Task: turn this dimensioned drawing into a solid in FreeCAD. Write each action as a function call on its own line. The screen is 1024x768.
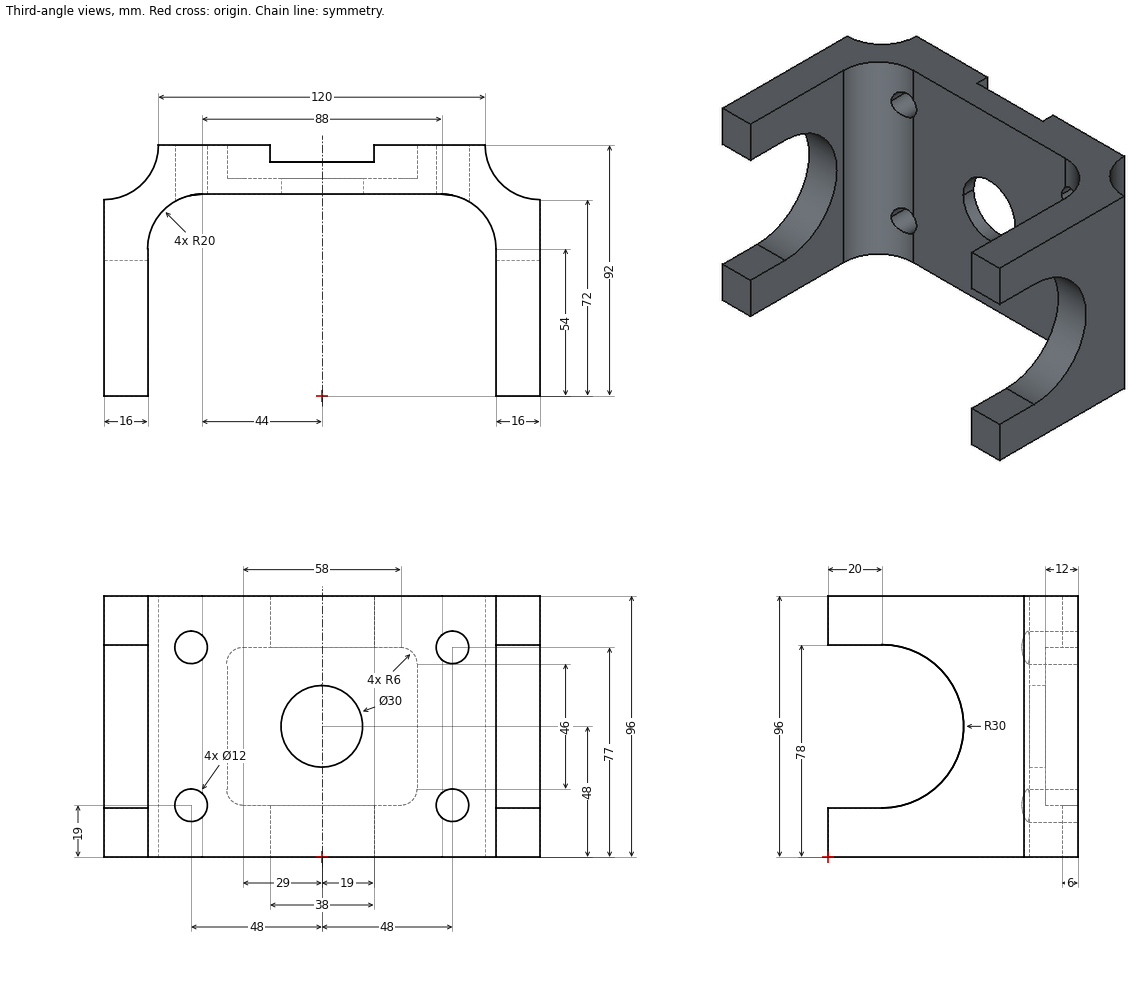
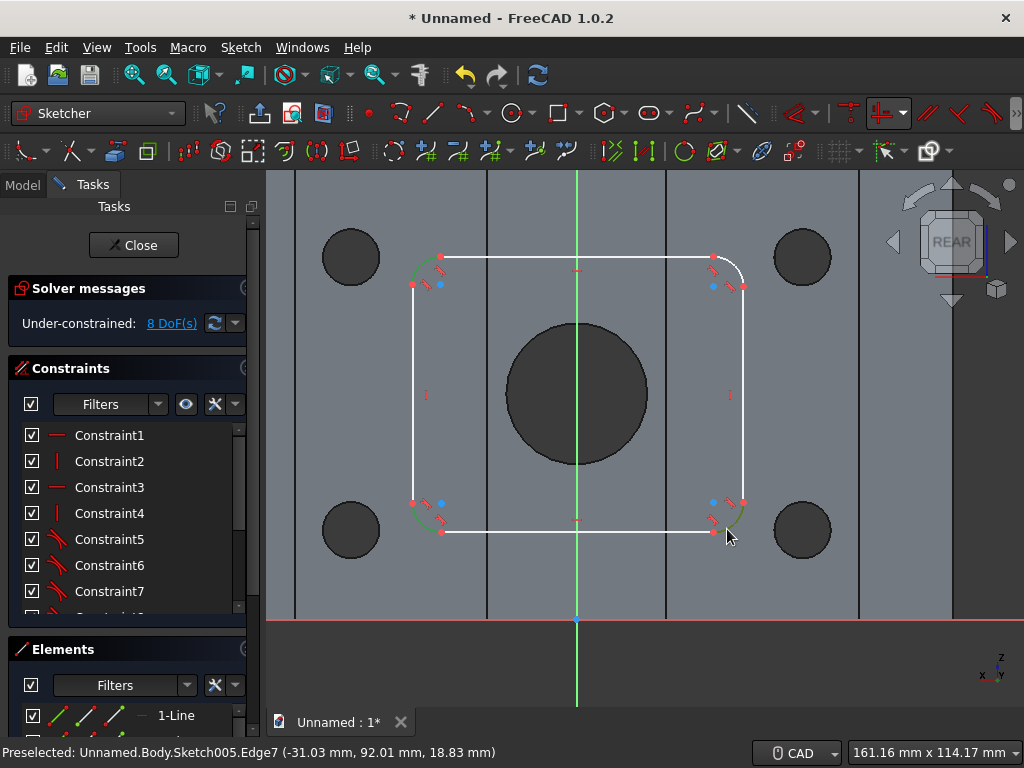
click(740, 273)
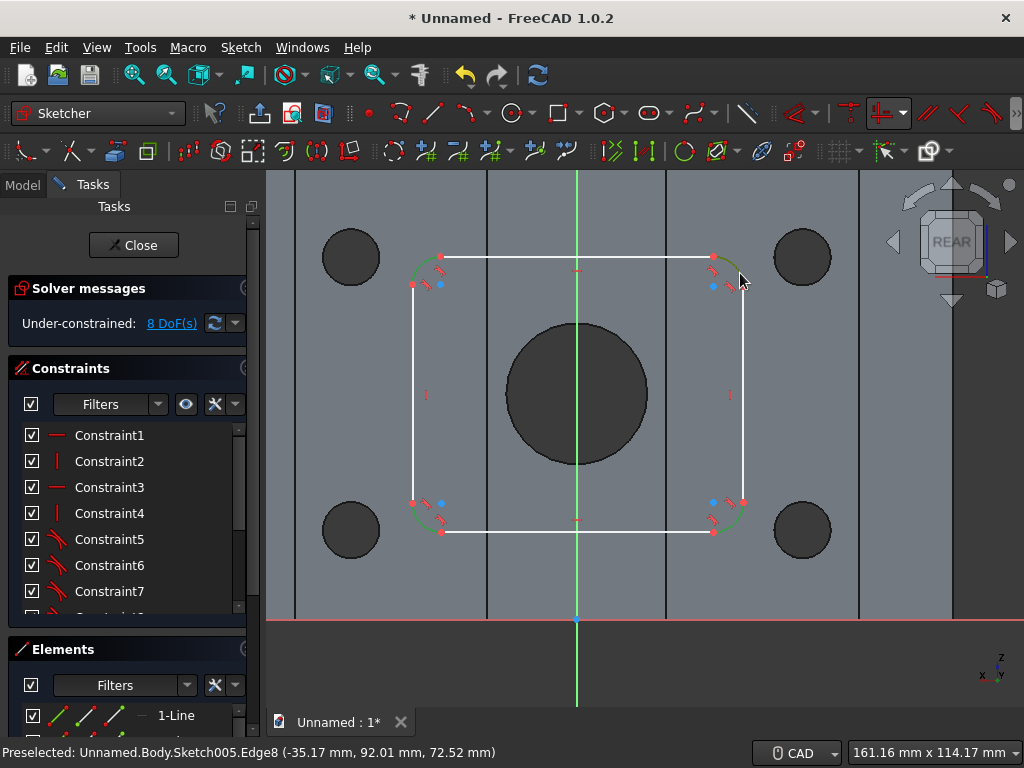
key(e)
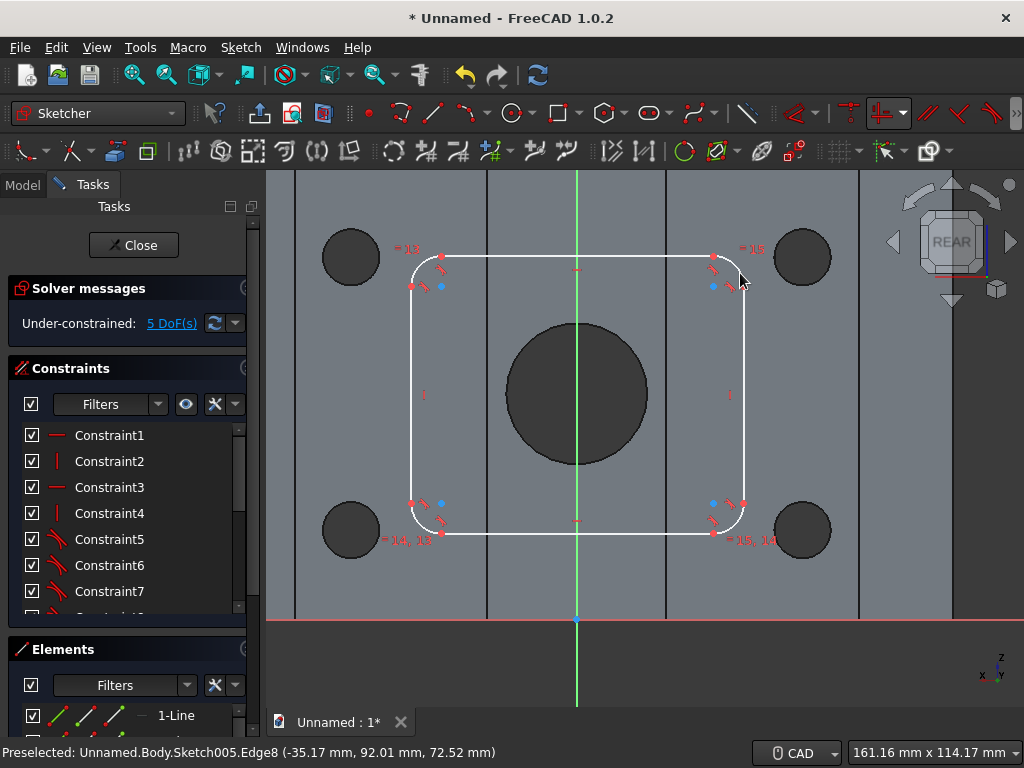
click(794, 114)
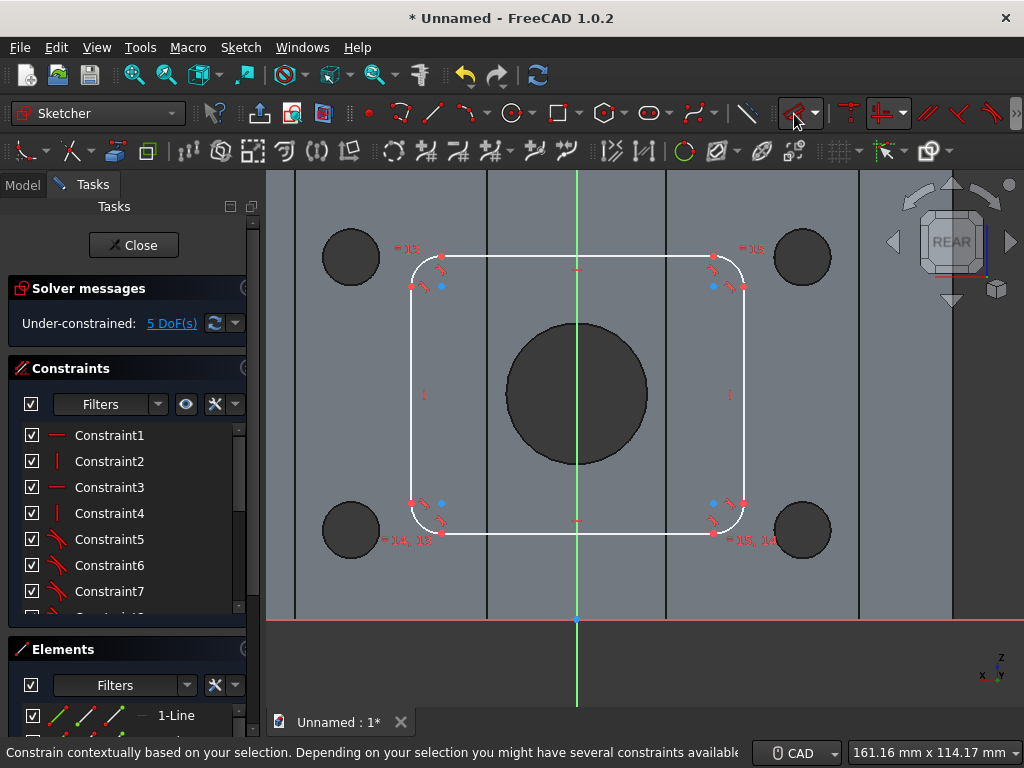
scroll(428, 259, up, 2)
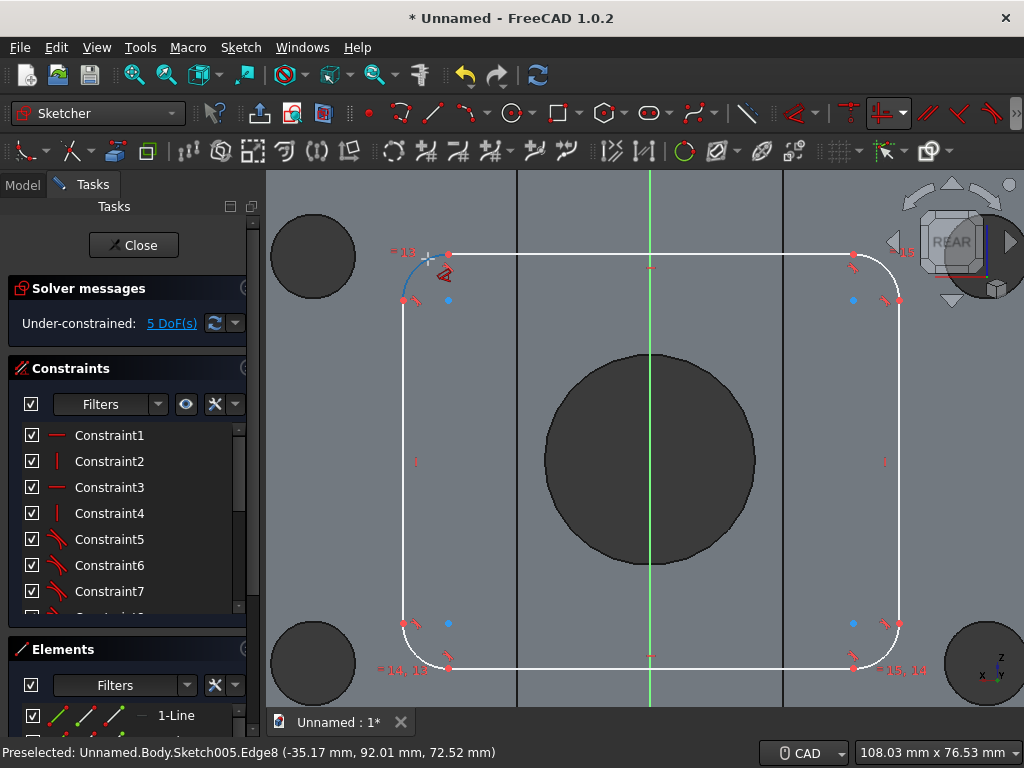
click(428, 259)
click(414, 230)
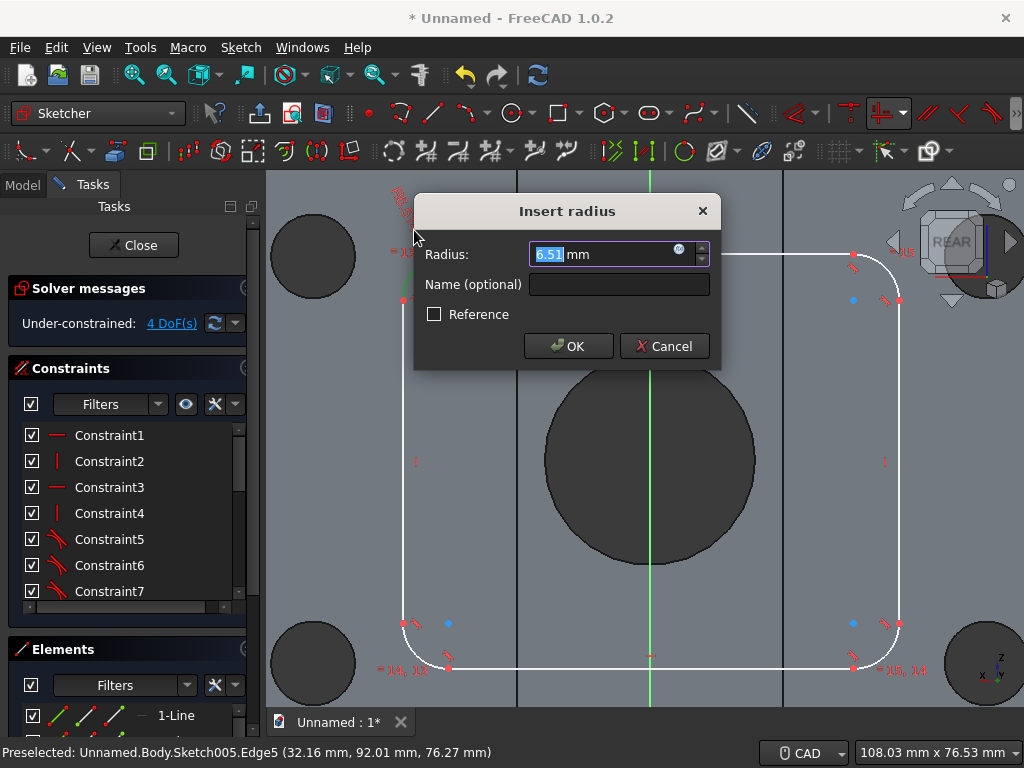
text(6)
key(Return)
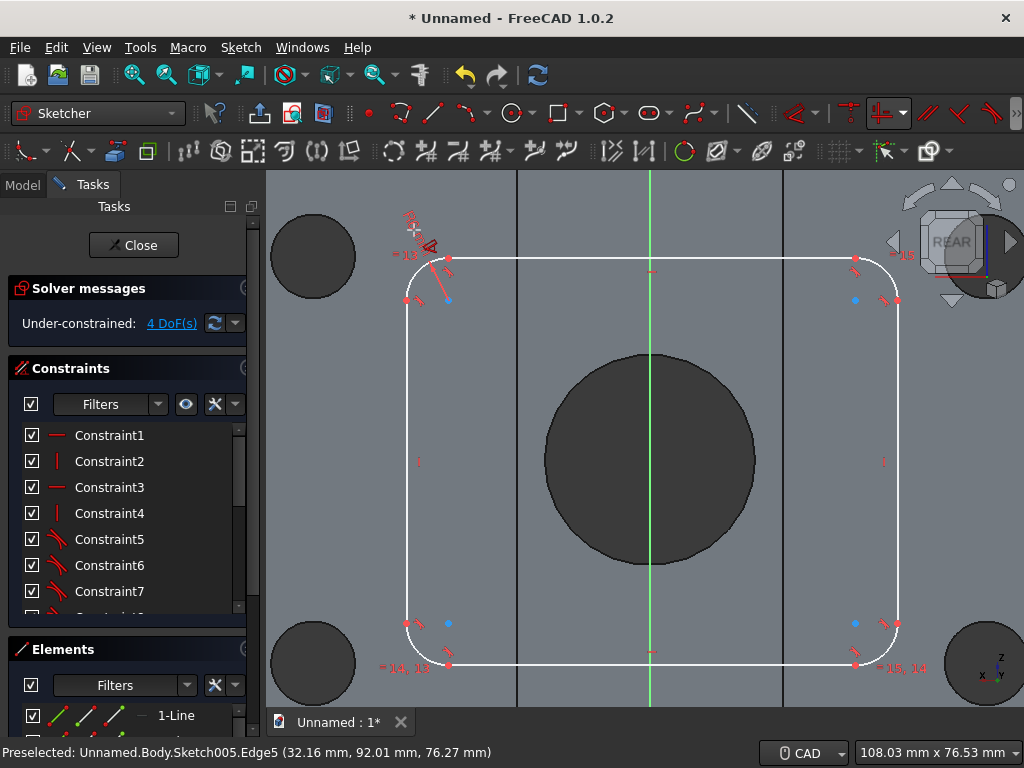
click(734, 258)
click(559, 224)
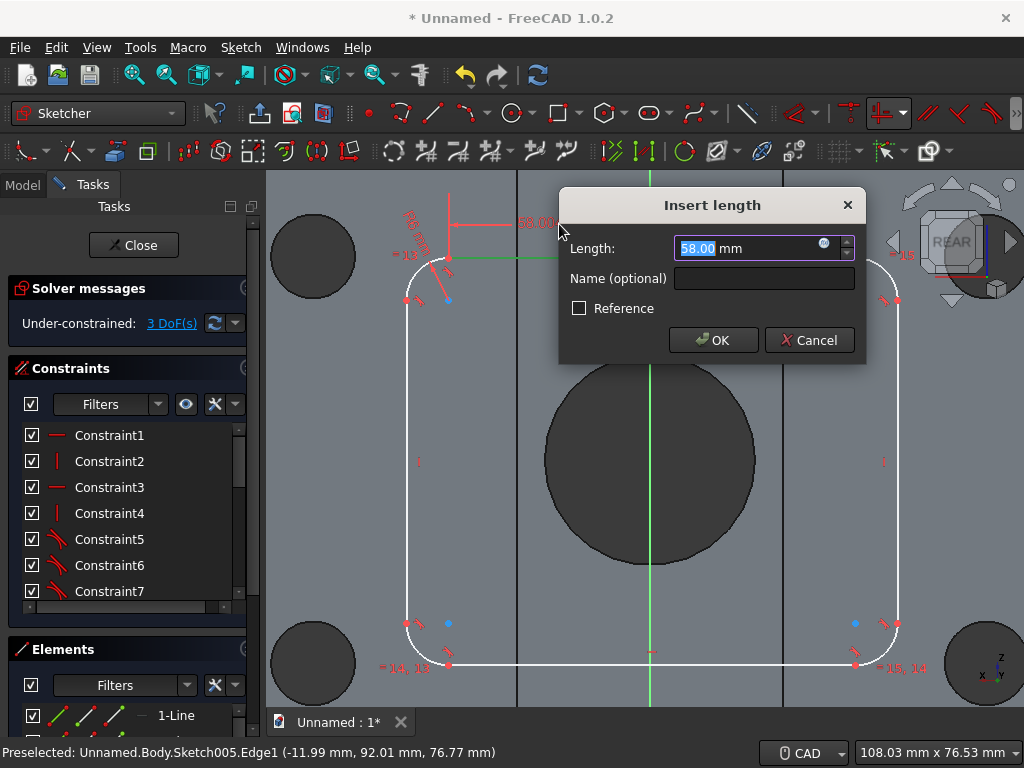
text(58)
key(Return)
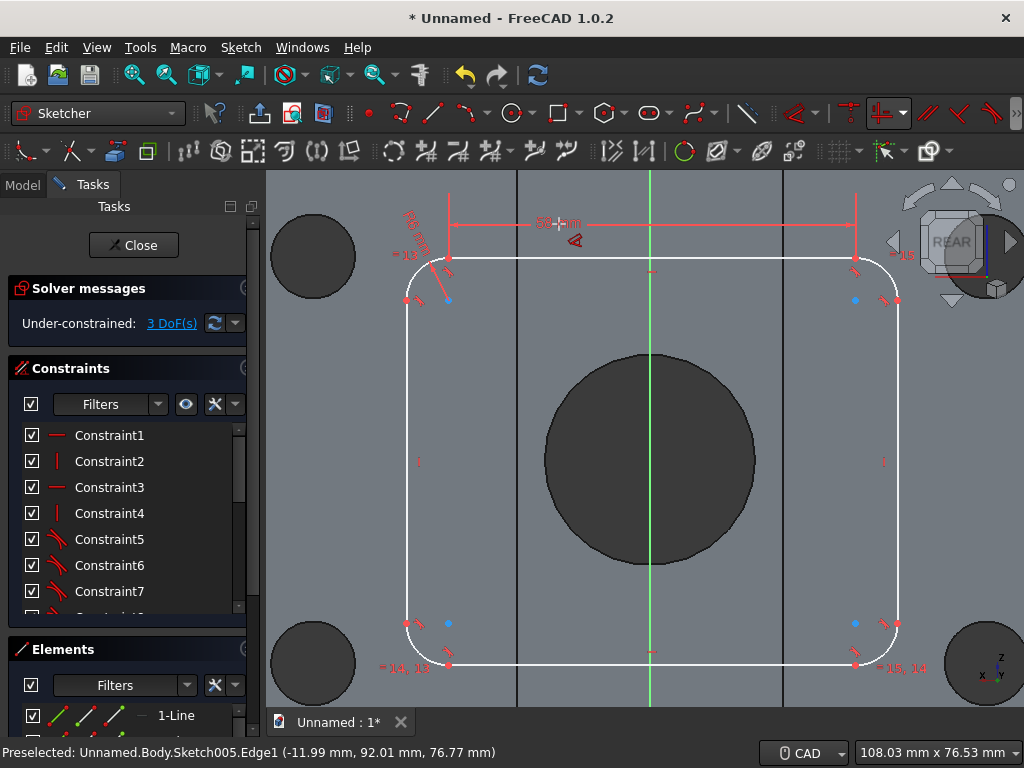
click(407, 397)
click(373, 462)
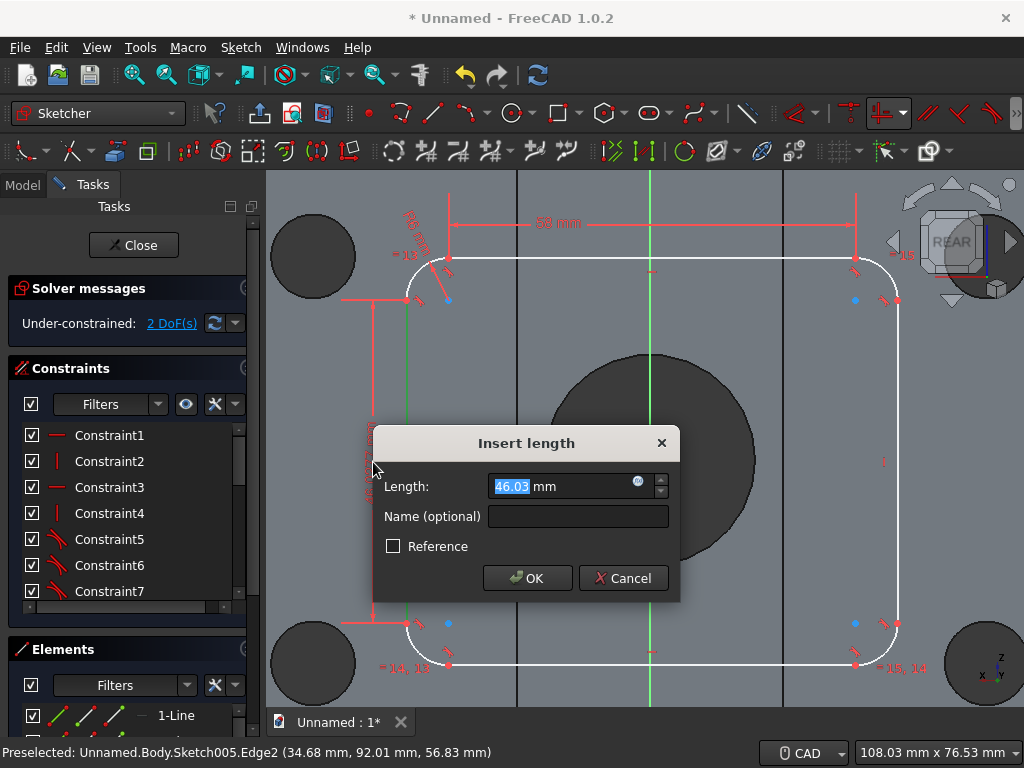
text(46)
key(Return)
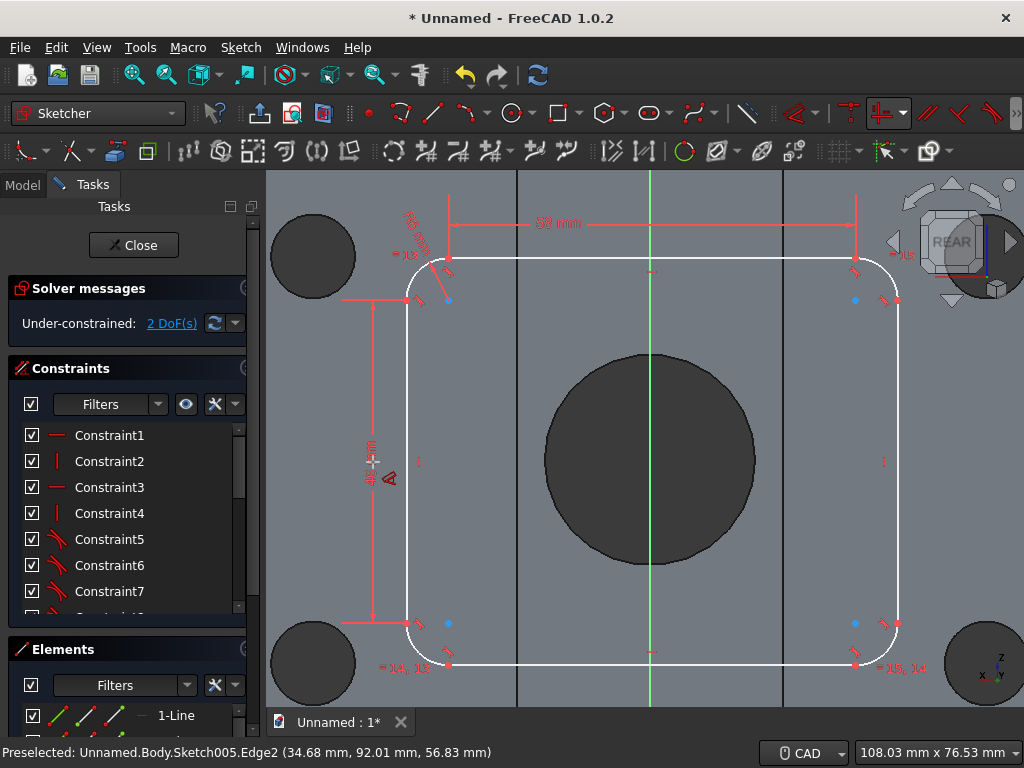
click(856, 258)
click(753, 224)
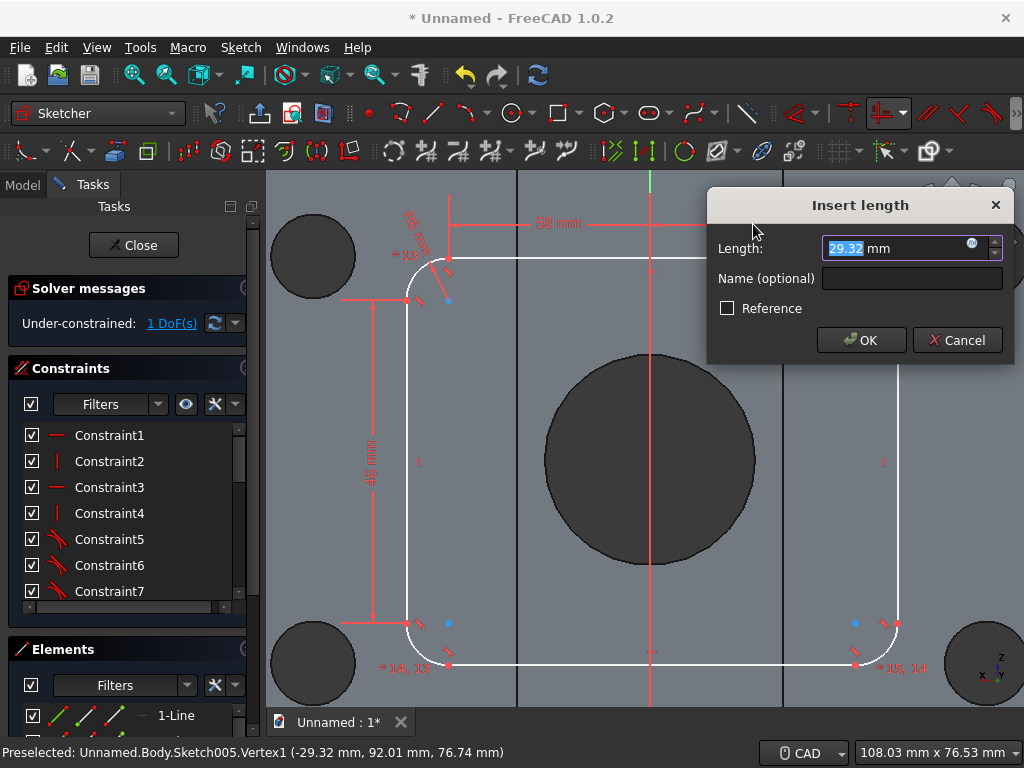
text(29)
key(Return)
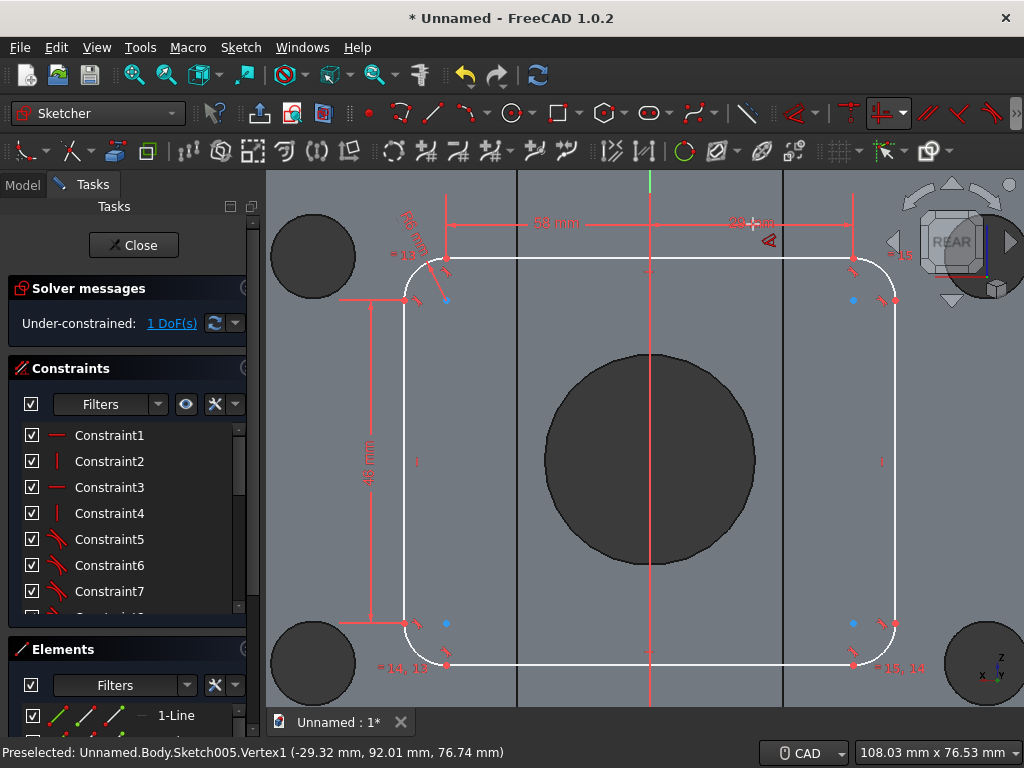
click(853, 258)
click(616, 469)